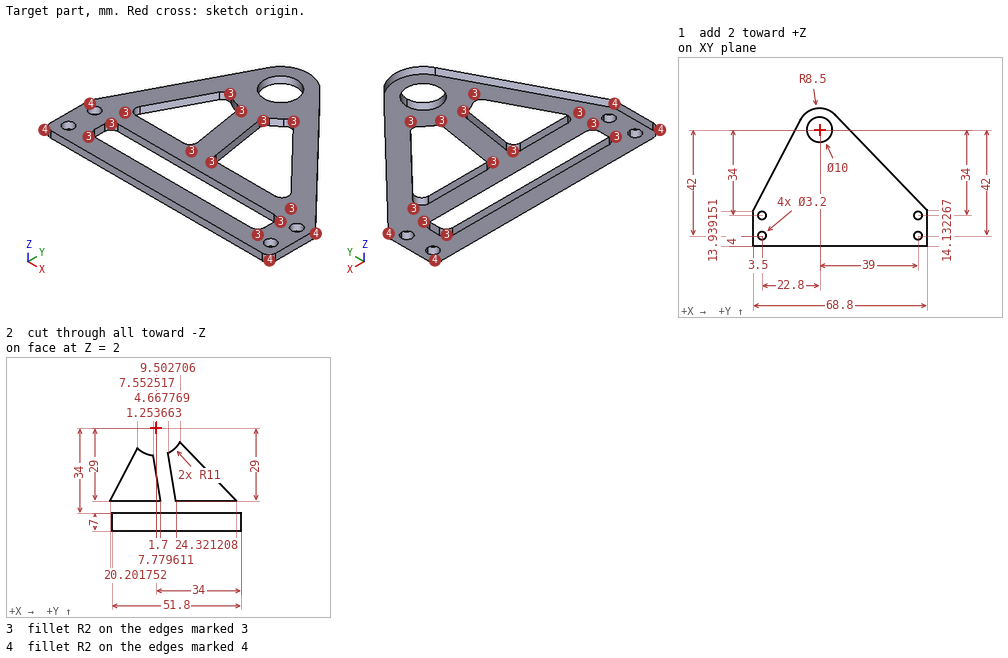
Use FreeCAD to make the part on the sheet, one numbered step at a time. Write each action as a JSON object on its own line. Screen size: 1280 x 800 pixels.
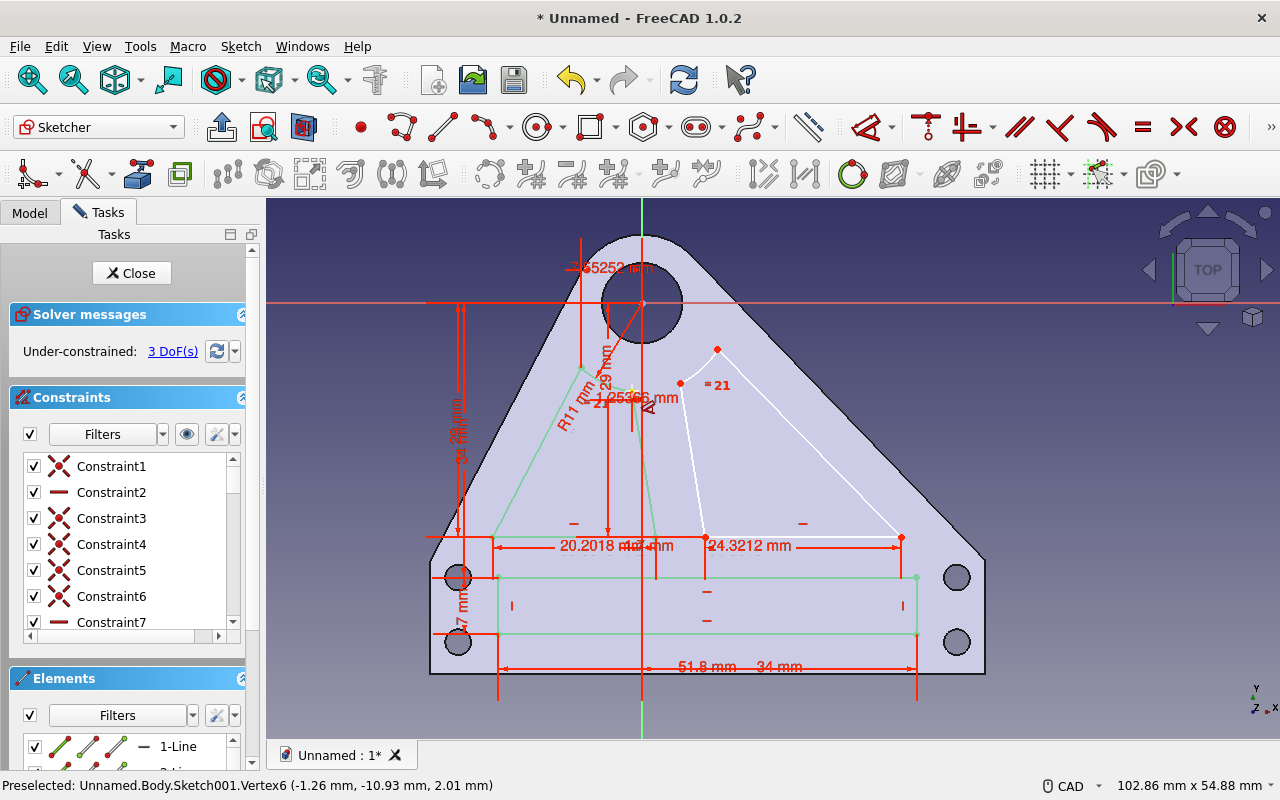
{"action": "left_click", "coordinate": [680, 383]}
{"action": "left_click", "coordinate": [661, 245]}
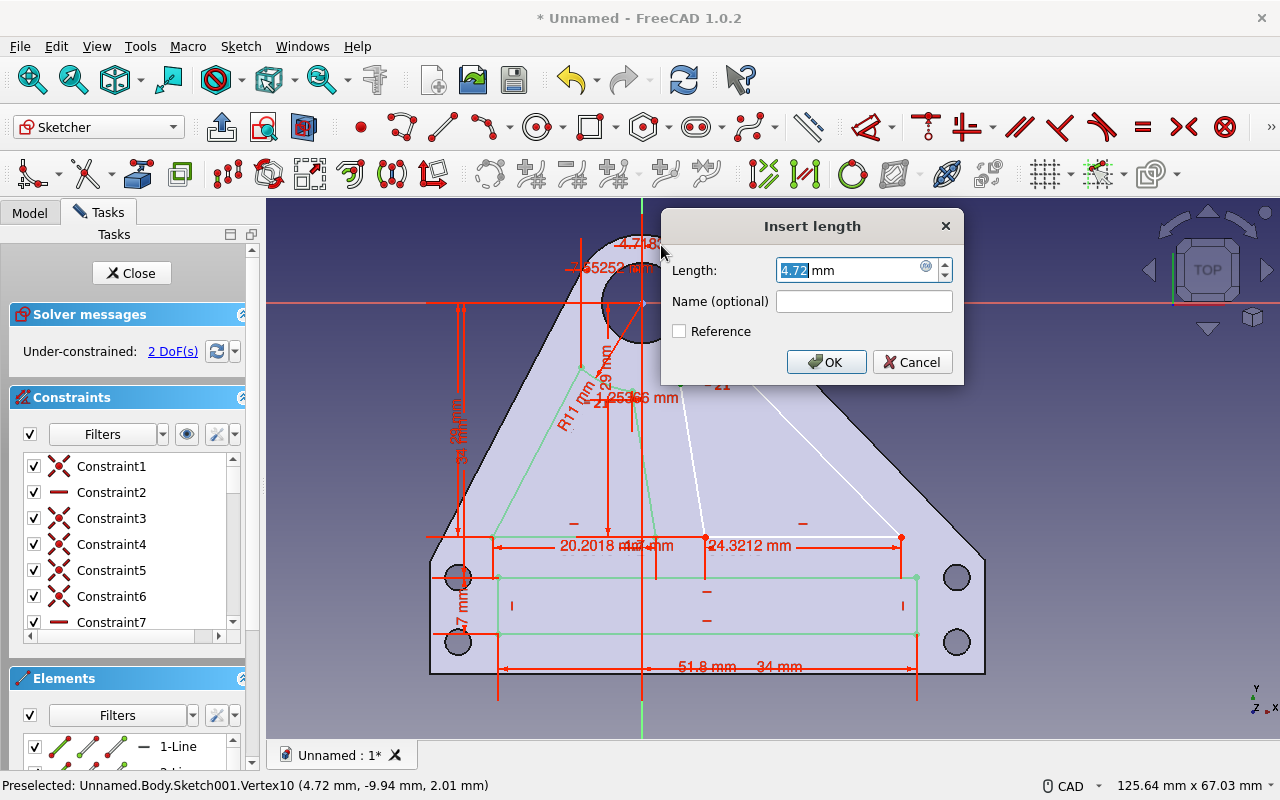
{"action": "type", "text": "4.667769"}
{"action": "key", "text": "Return"}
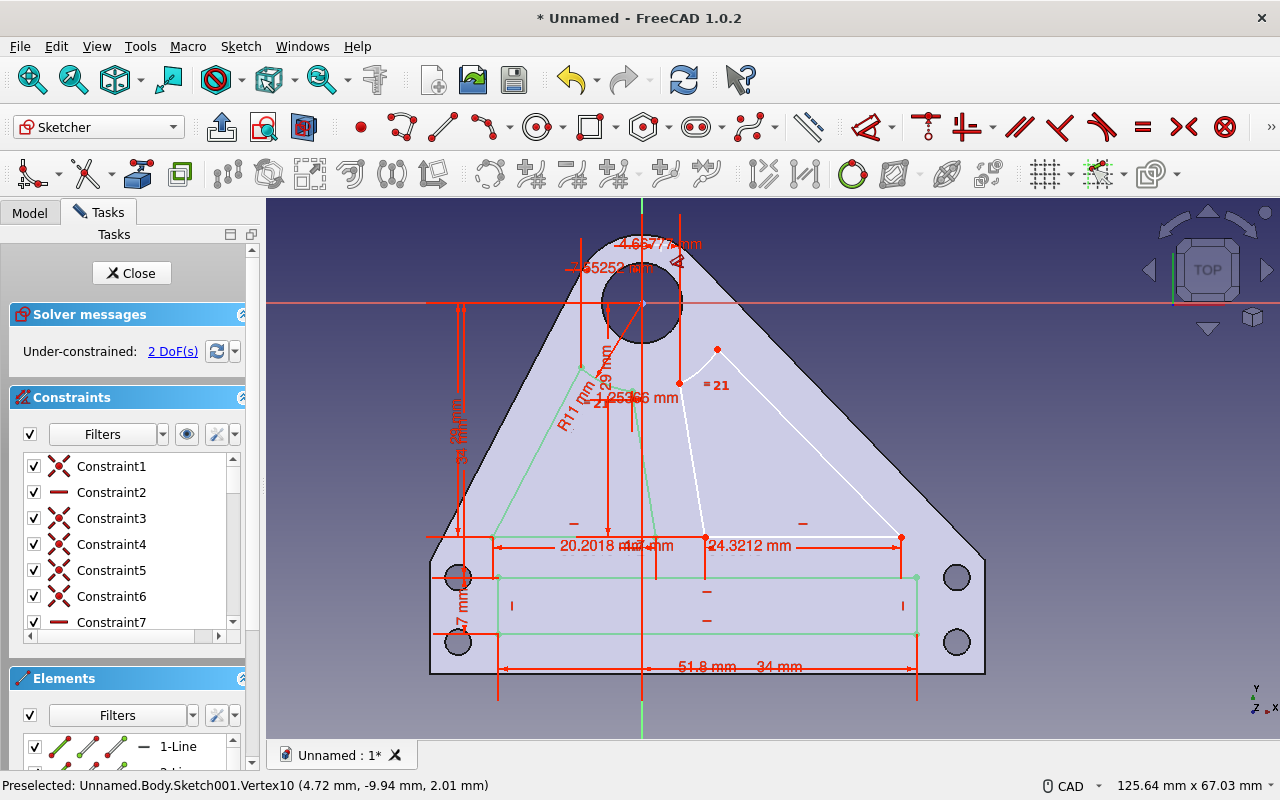
{"action": "left_click", "coordinate": [705, 537]}
{"action": "left_click", "coordinate": [688, 269]}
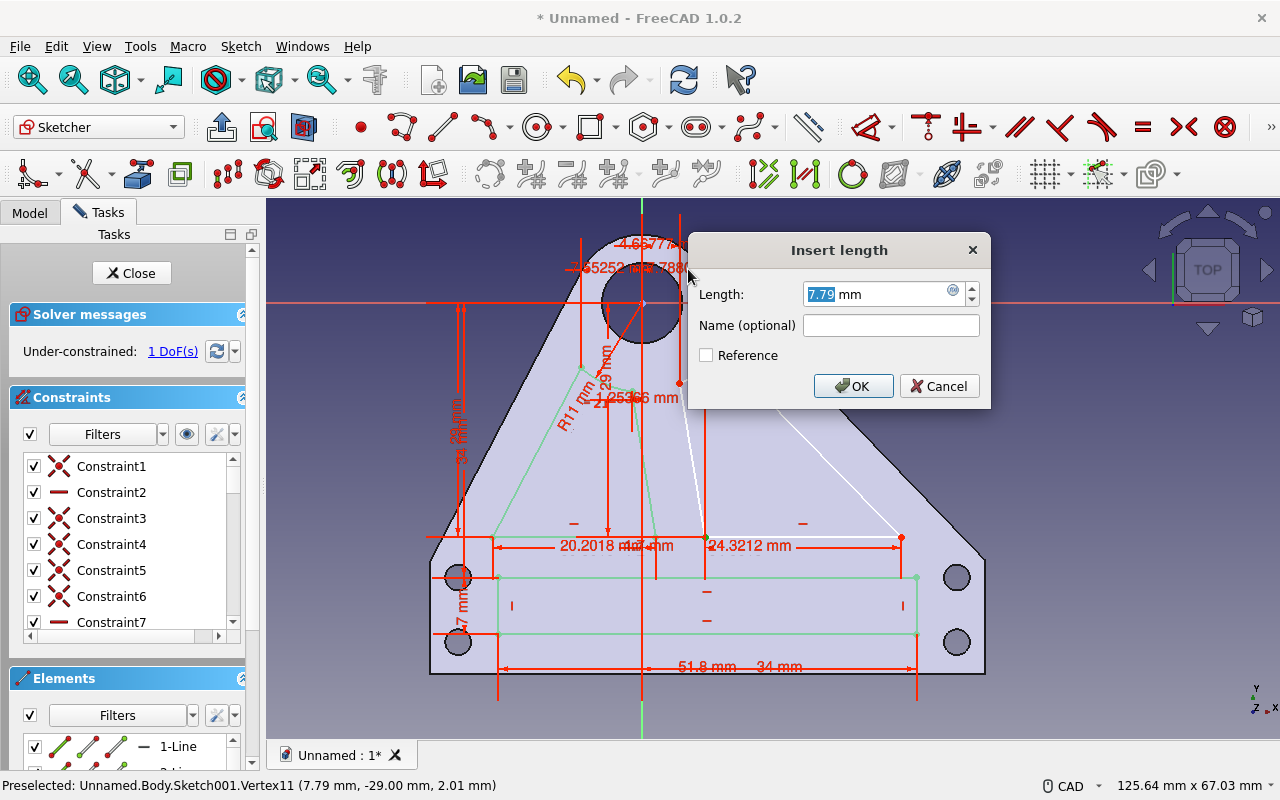
{"action": "type", "text": "7.779611"}
{"action": "key", "text": "Return"}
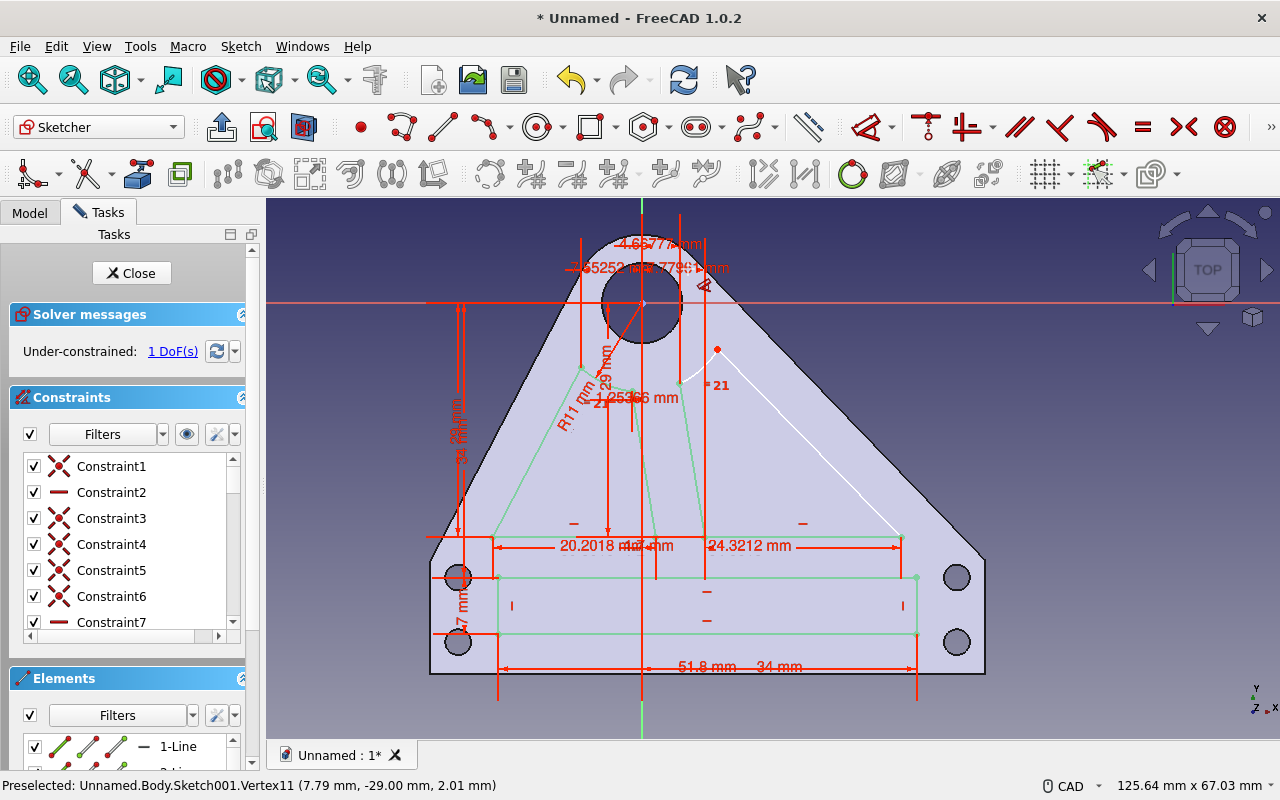
{"action": "left_click", "coordinate": [718, 349]}
{"action": "left_click", "coordinate": [663, 431]}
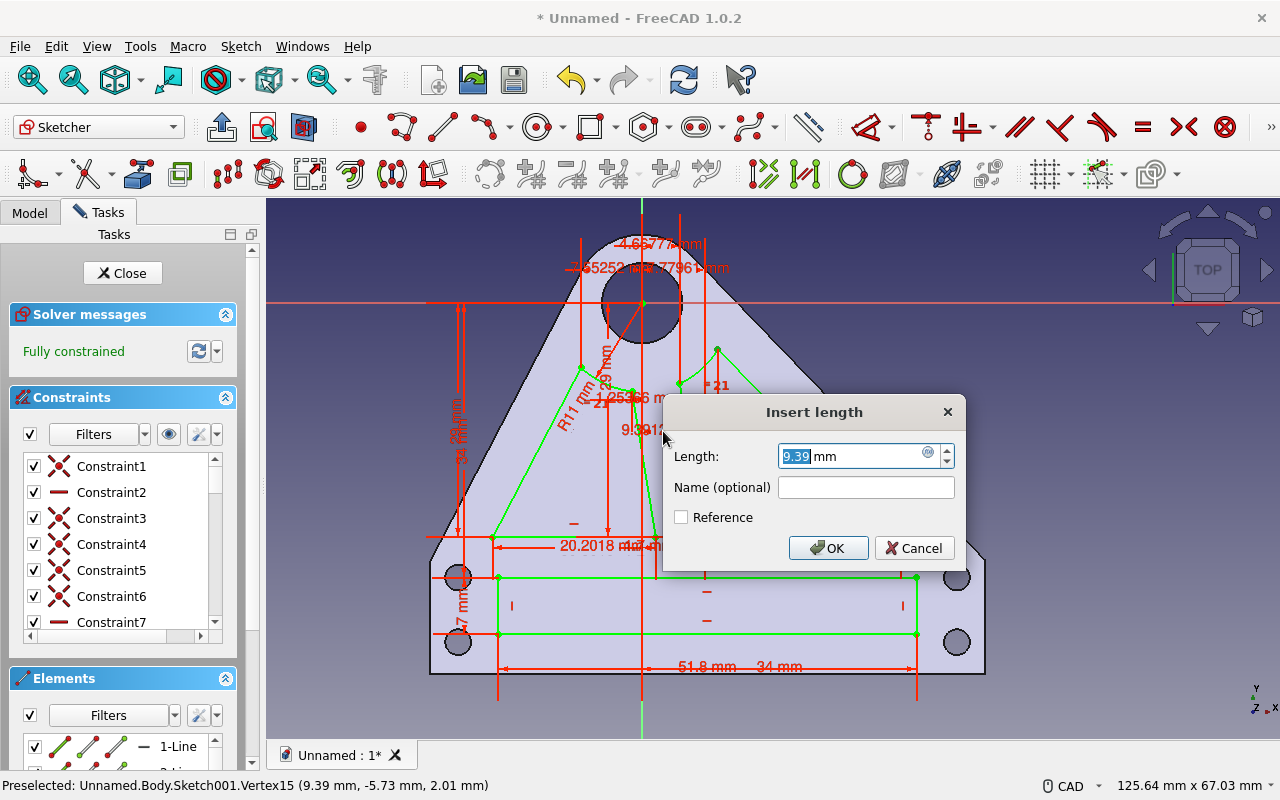
{"action": "type", "text": "9.502706"}
{"action": "key", "text": "Return"}
{"action": "key", "text": "Escape"}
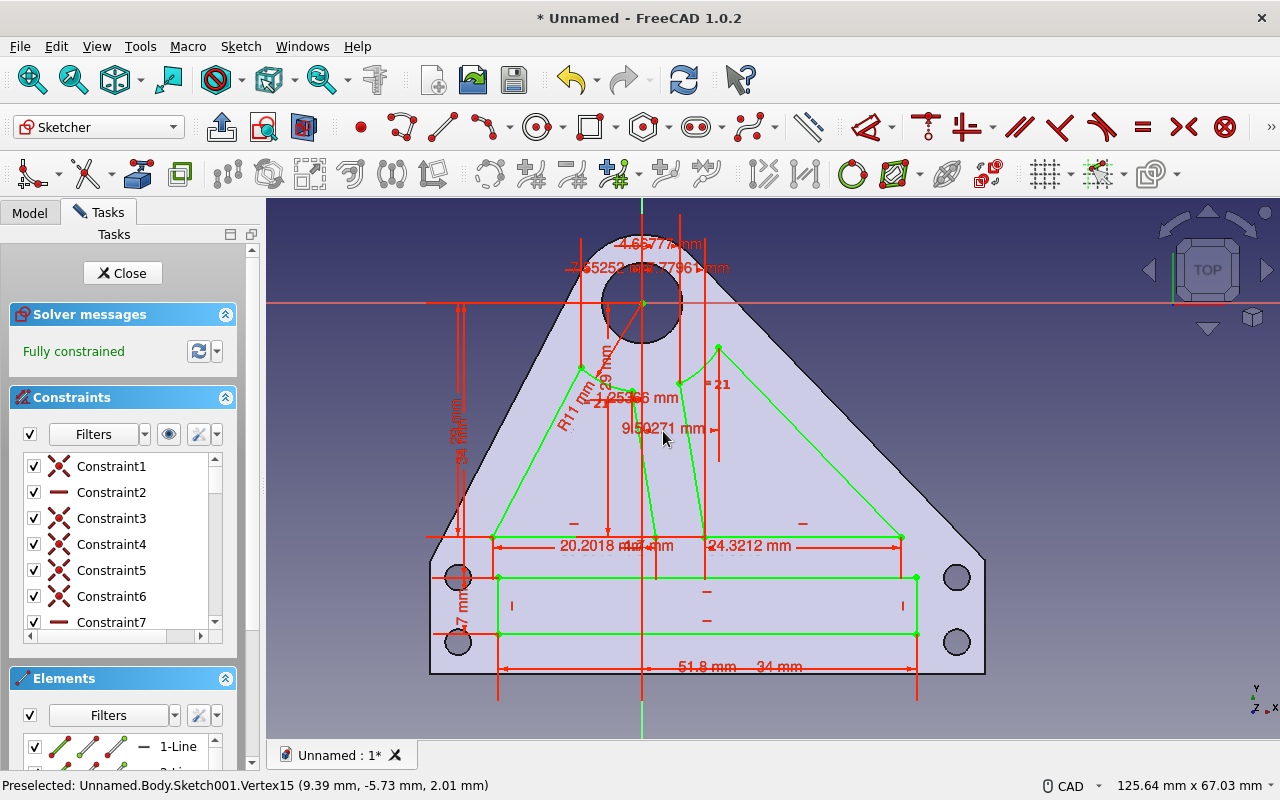
{"action": "left_click", "coordinate": [123, 273]}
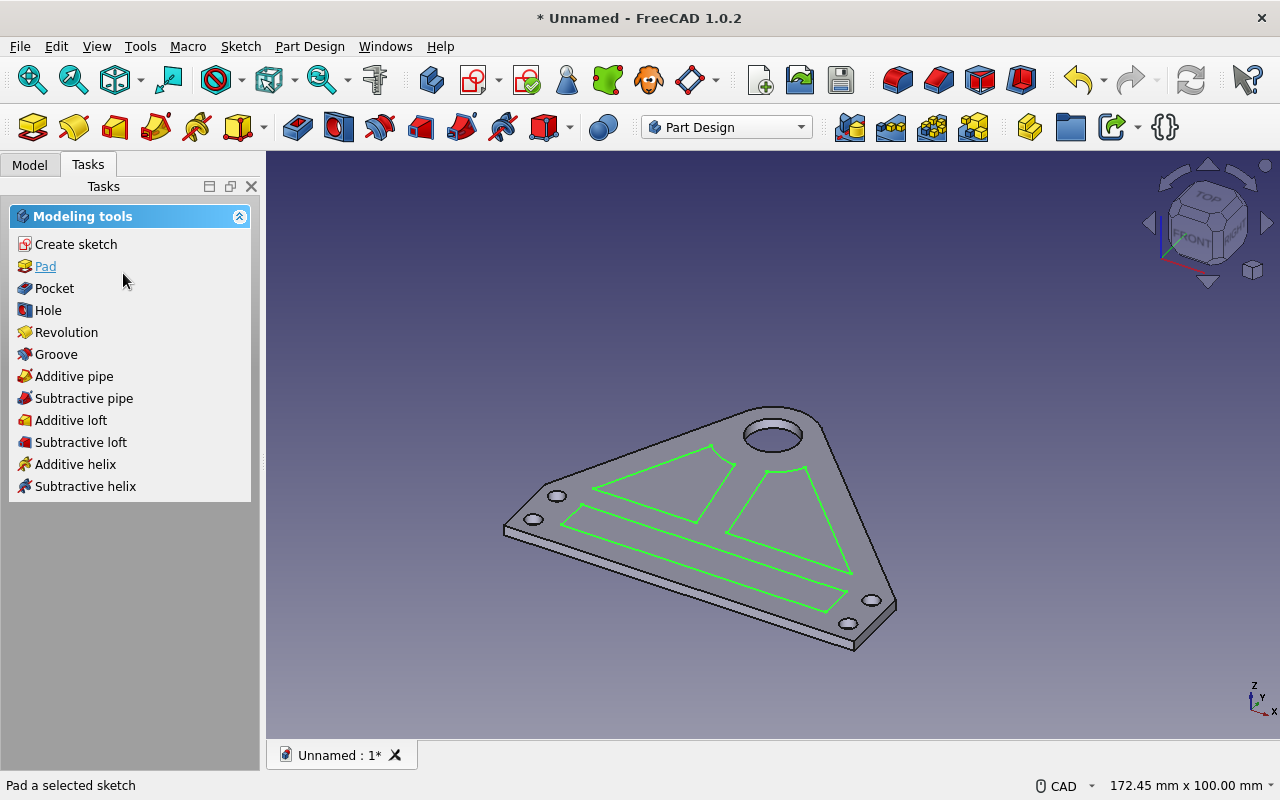
{"action": "left_click", "coordinate": [298, 128]}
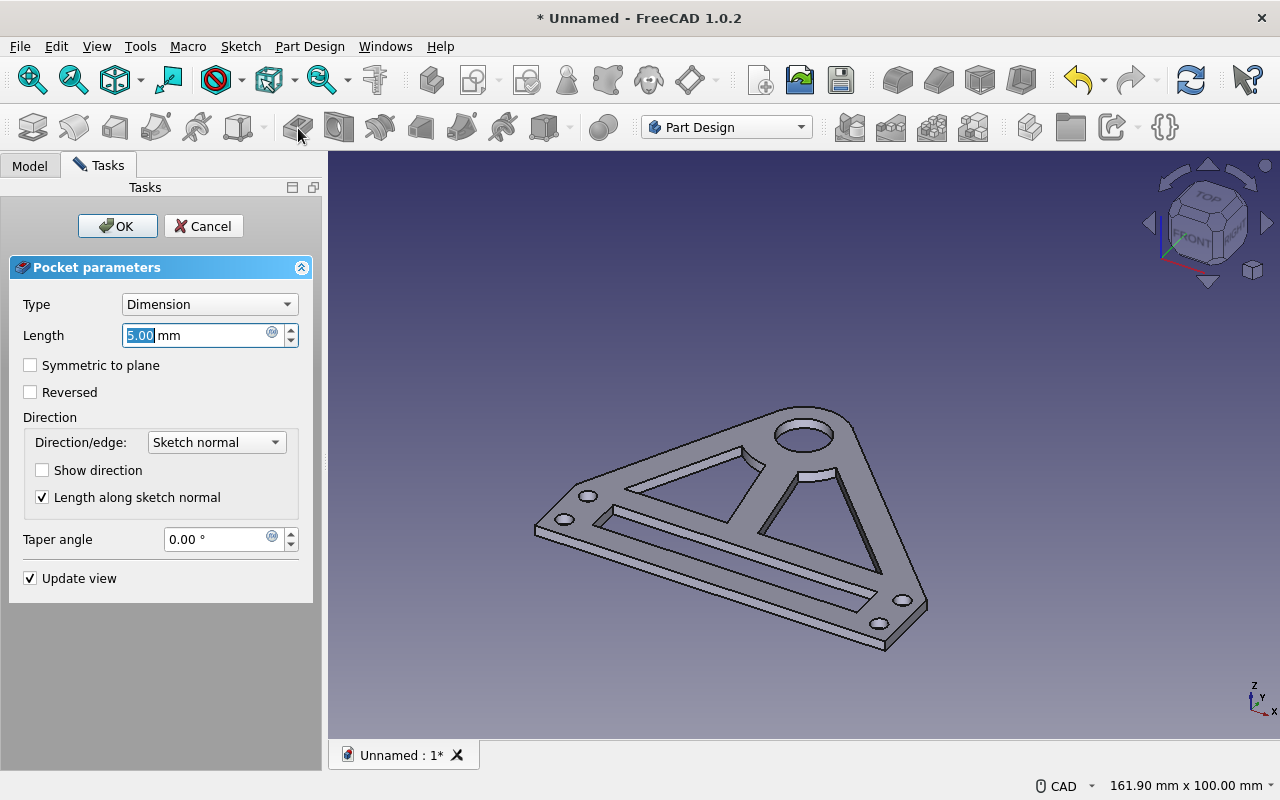
{"action": "left_click", "coordinate": [210, 304]}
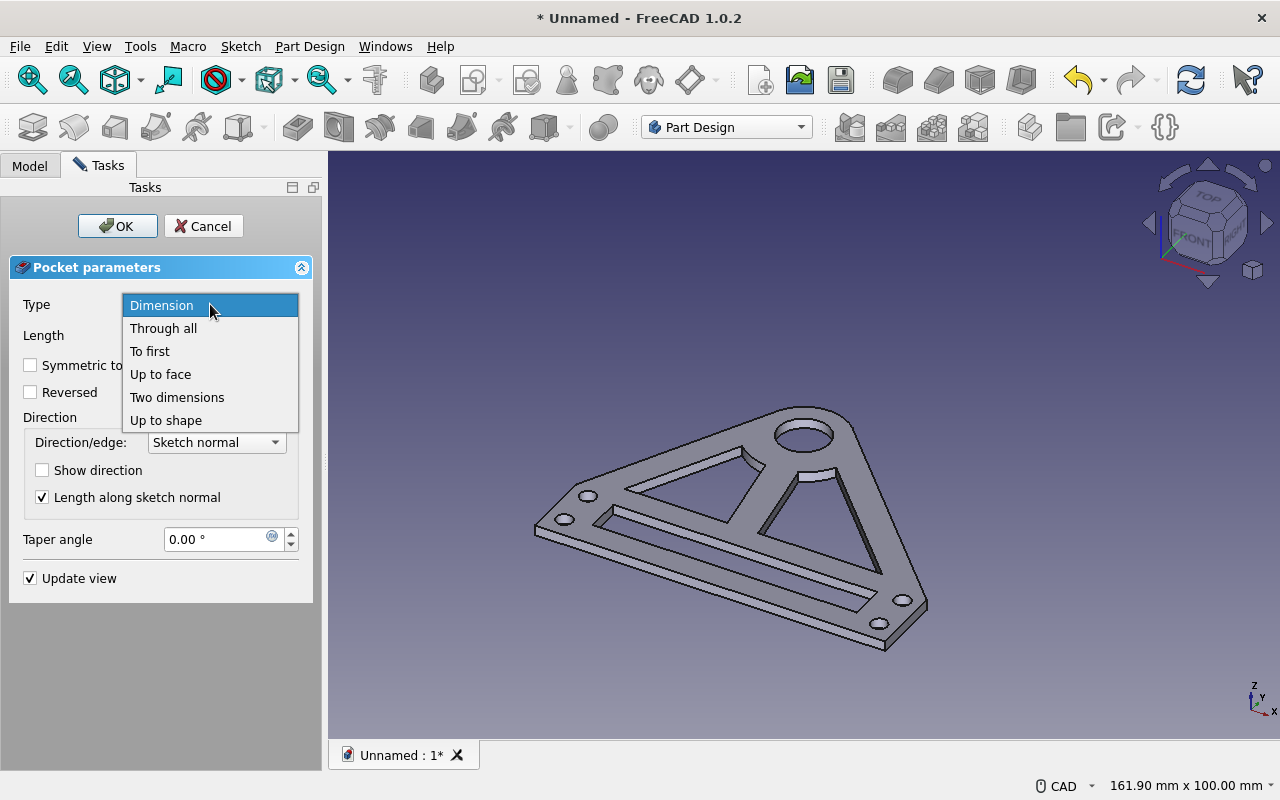
{"action": "left_click", "coordinate": [208, 328]}